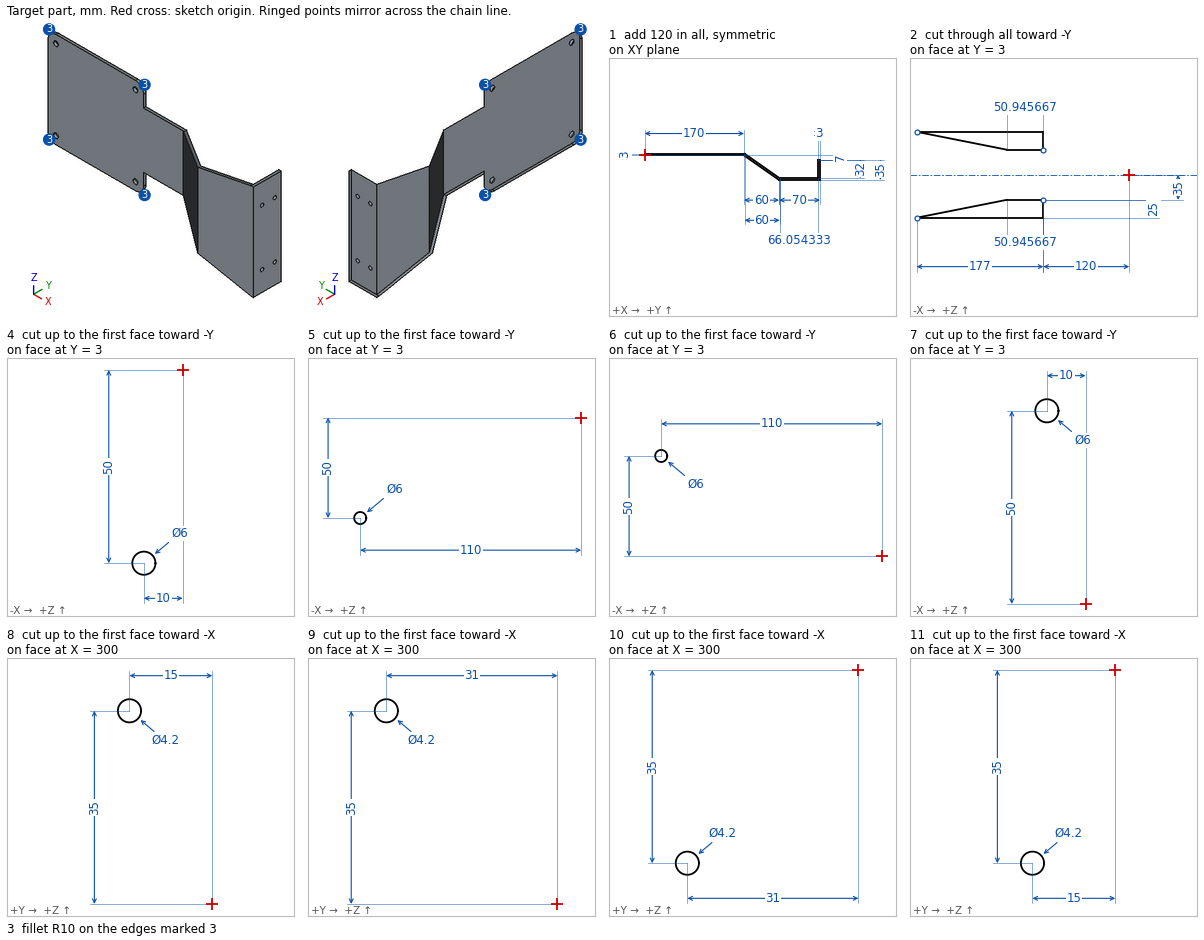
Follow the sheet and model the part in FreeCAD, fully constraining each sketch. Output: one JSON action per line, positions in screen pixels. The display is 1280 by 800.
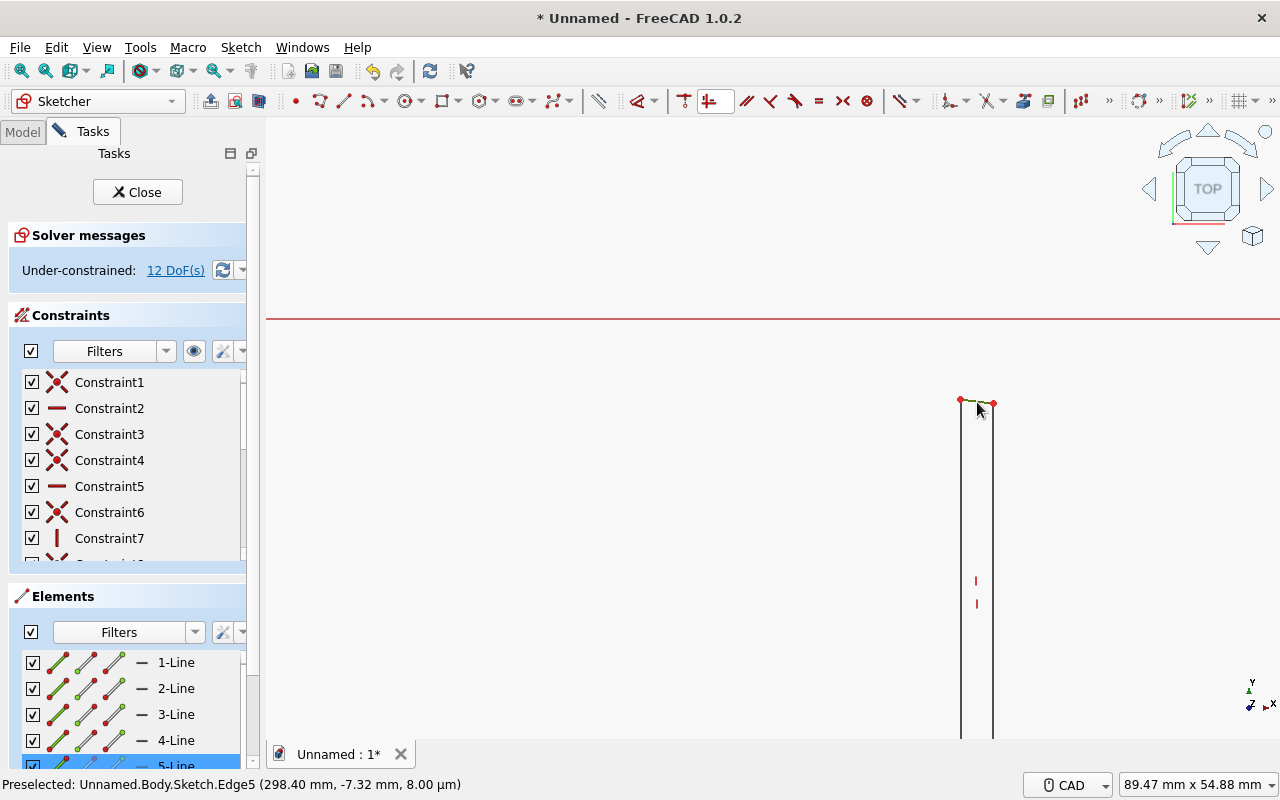
{"action": "left_click", "coordinate": [728, 102]}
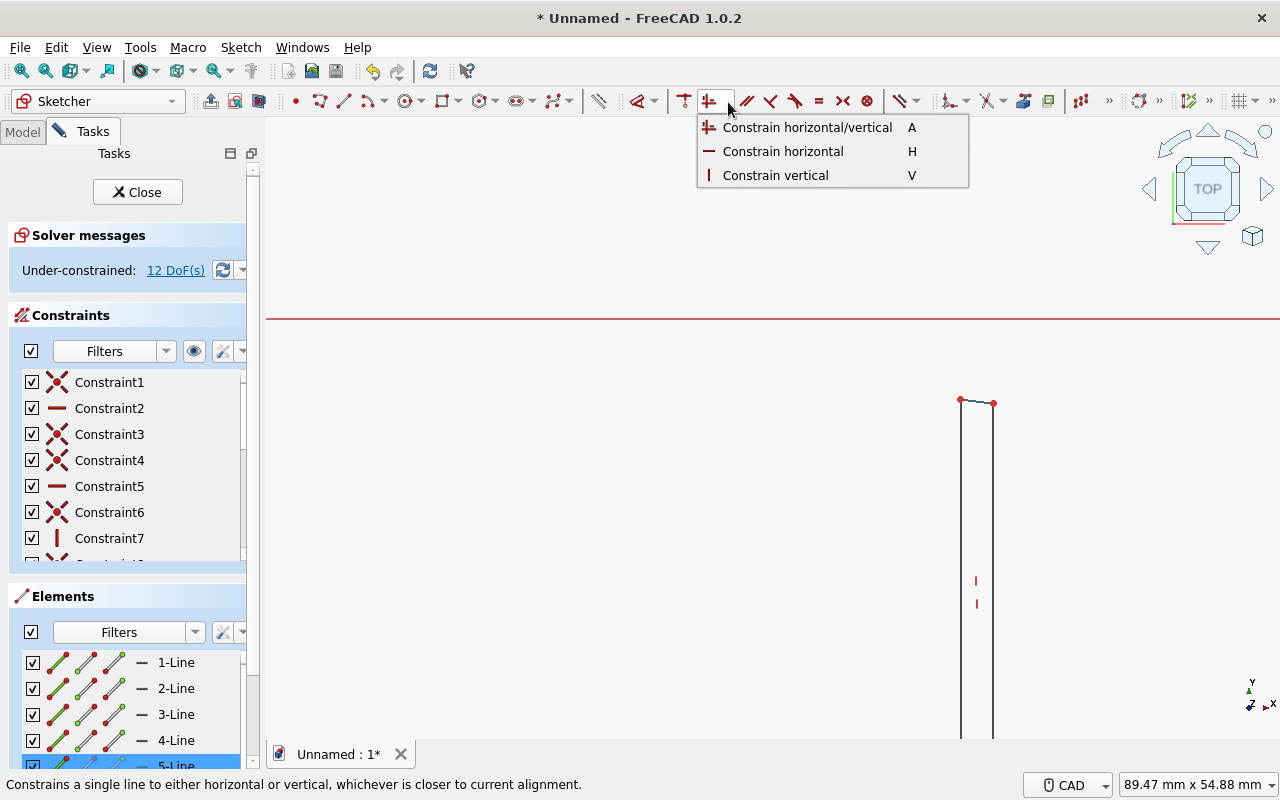
{"action": "left_click", "coordinate": [833, 151]}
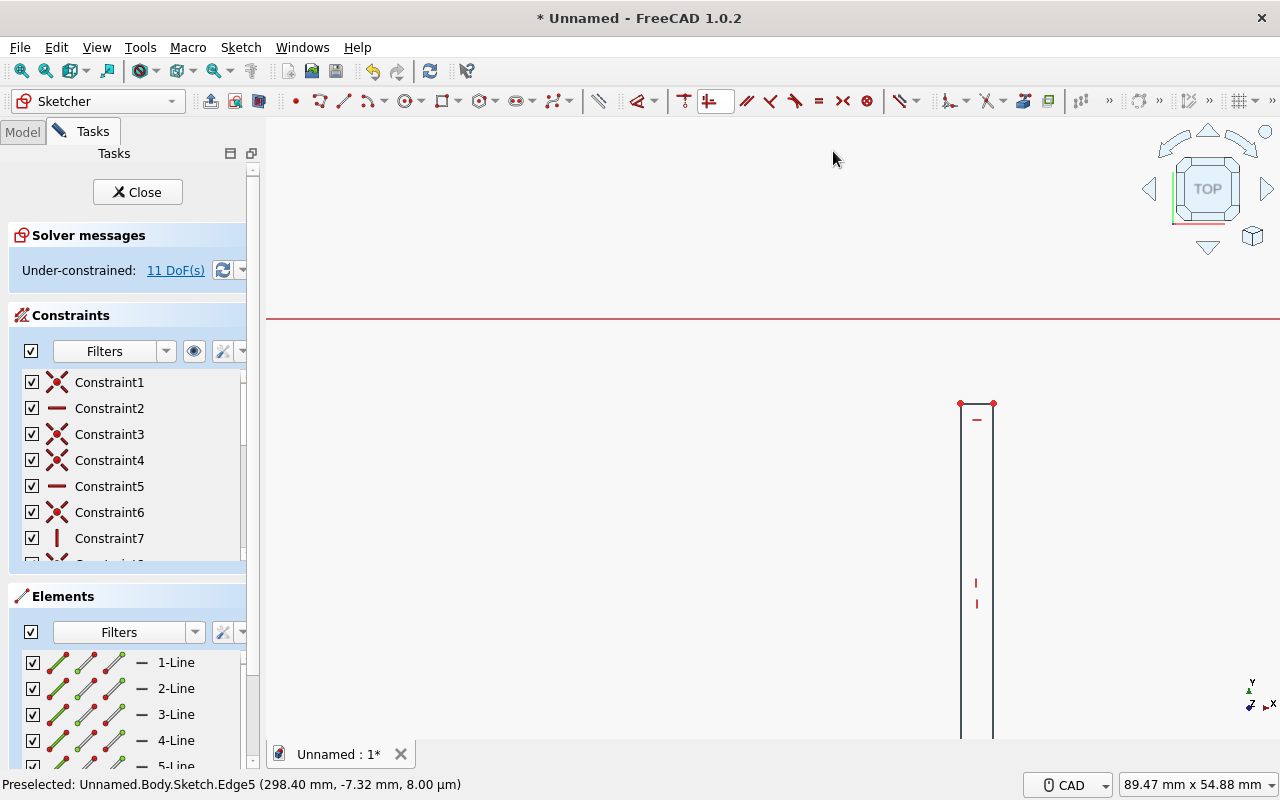
{"action": "scroll", "coordinate": [984, 406], "scroll_direction": "down", "scroll_amount": 9}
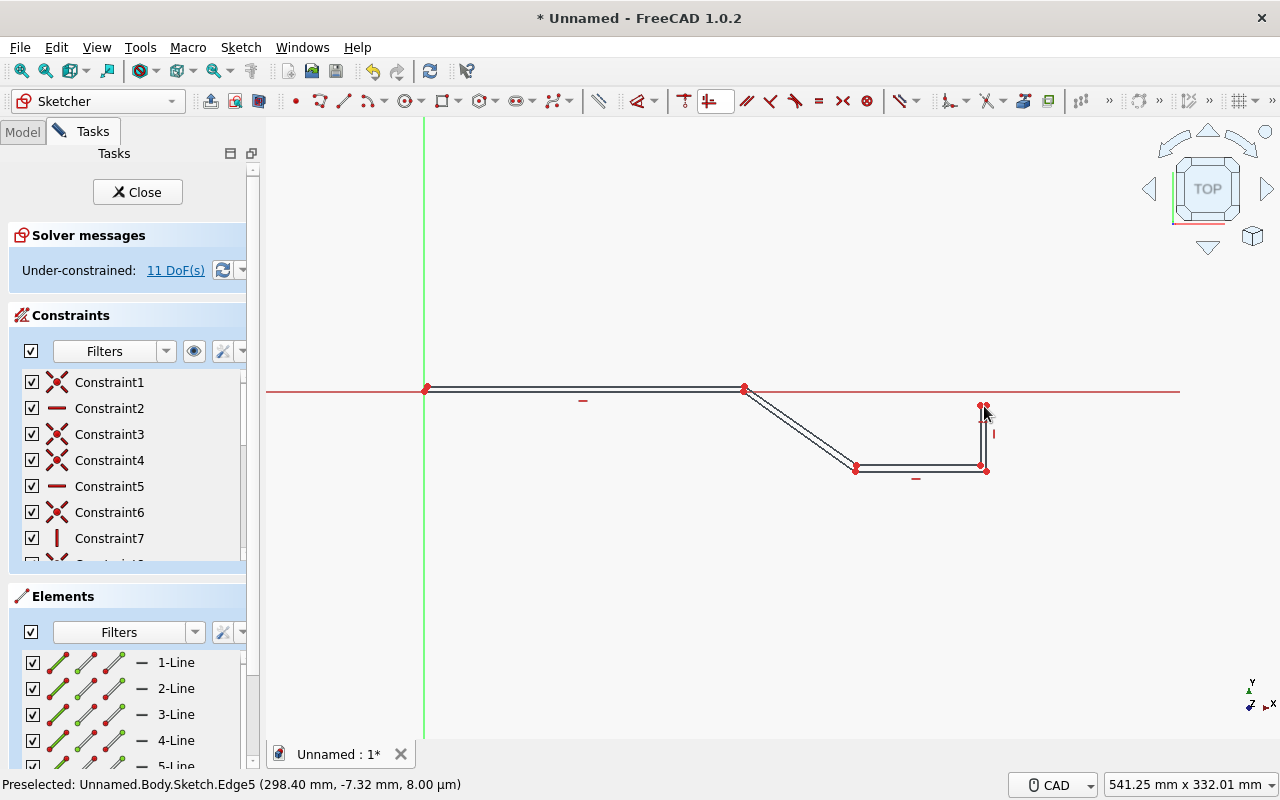
{"action": "scroll", "coordinate": [426, 388], "scroll_direction": "up", "scroll_amount": 11}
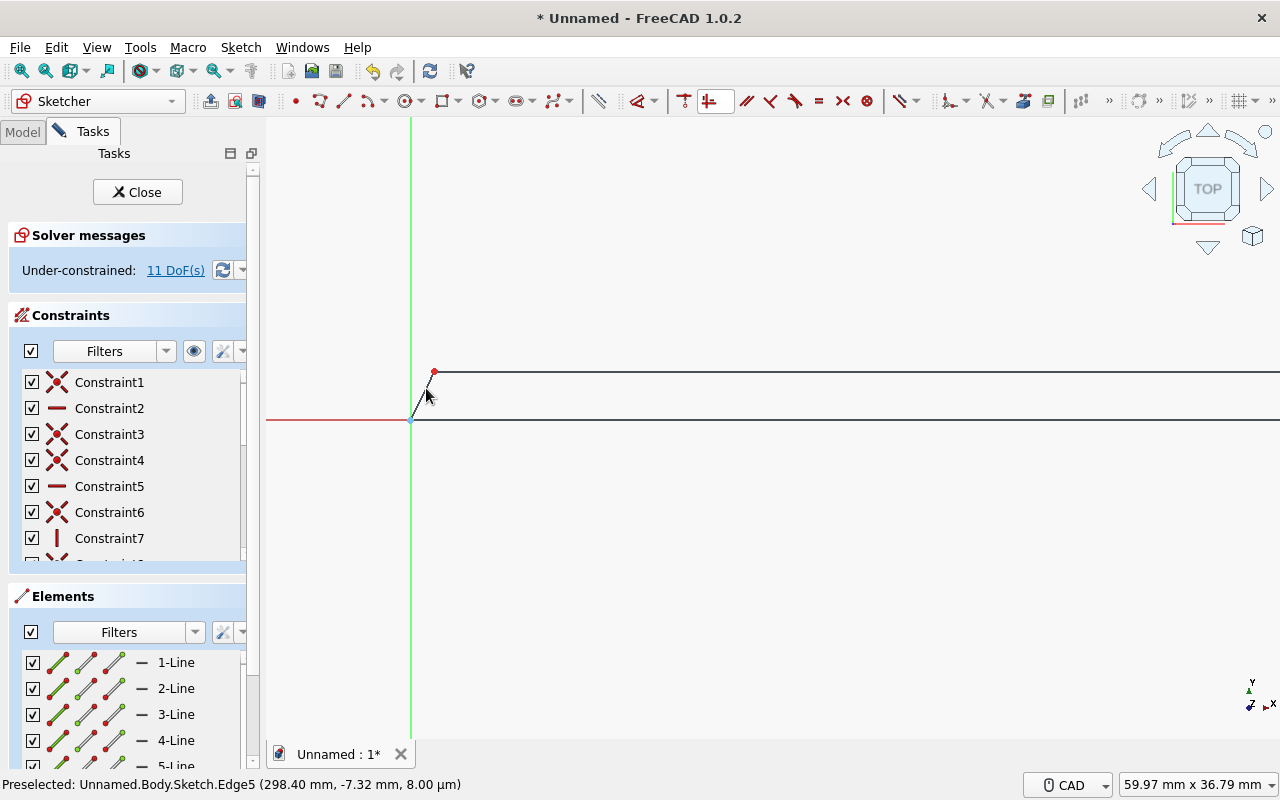
{"action": "left_click", "coordinate": [427, 386]}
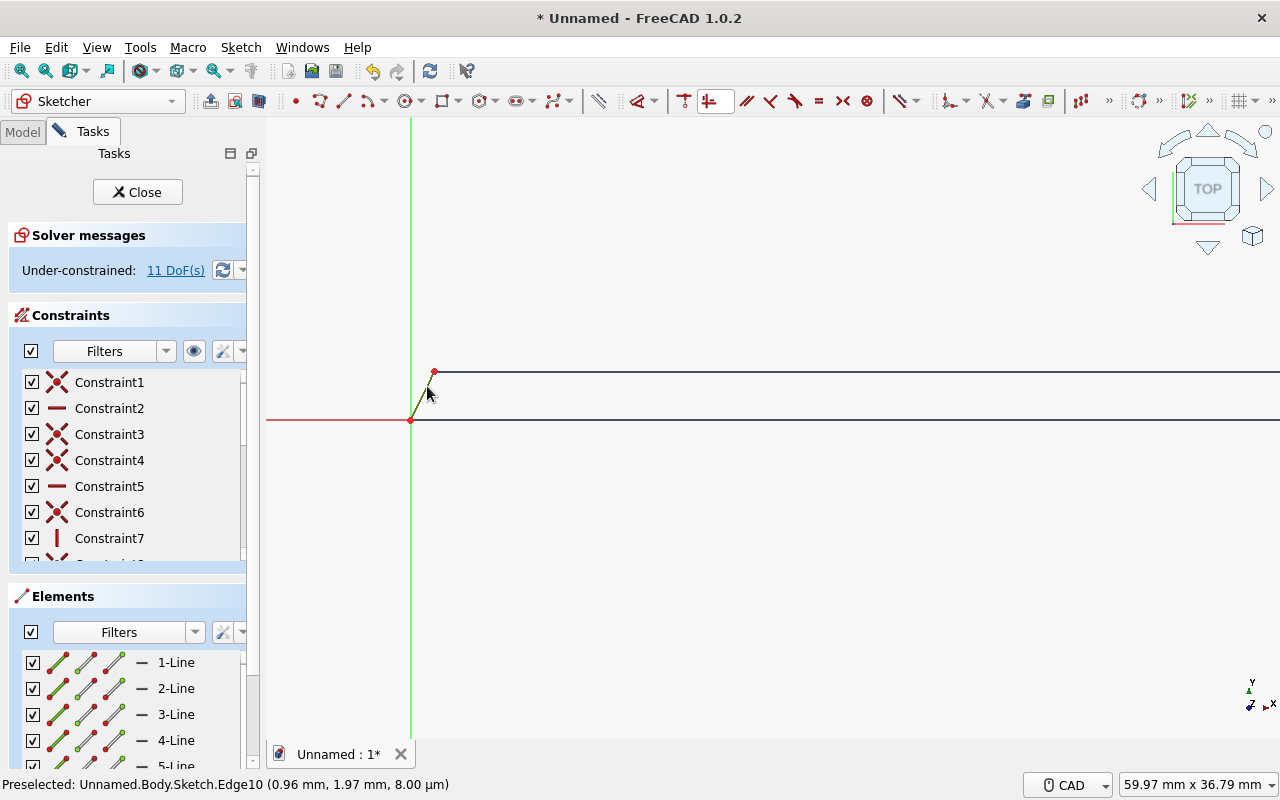
{"action": "left_click", "coordinate": [728, 102]}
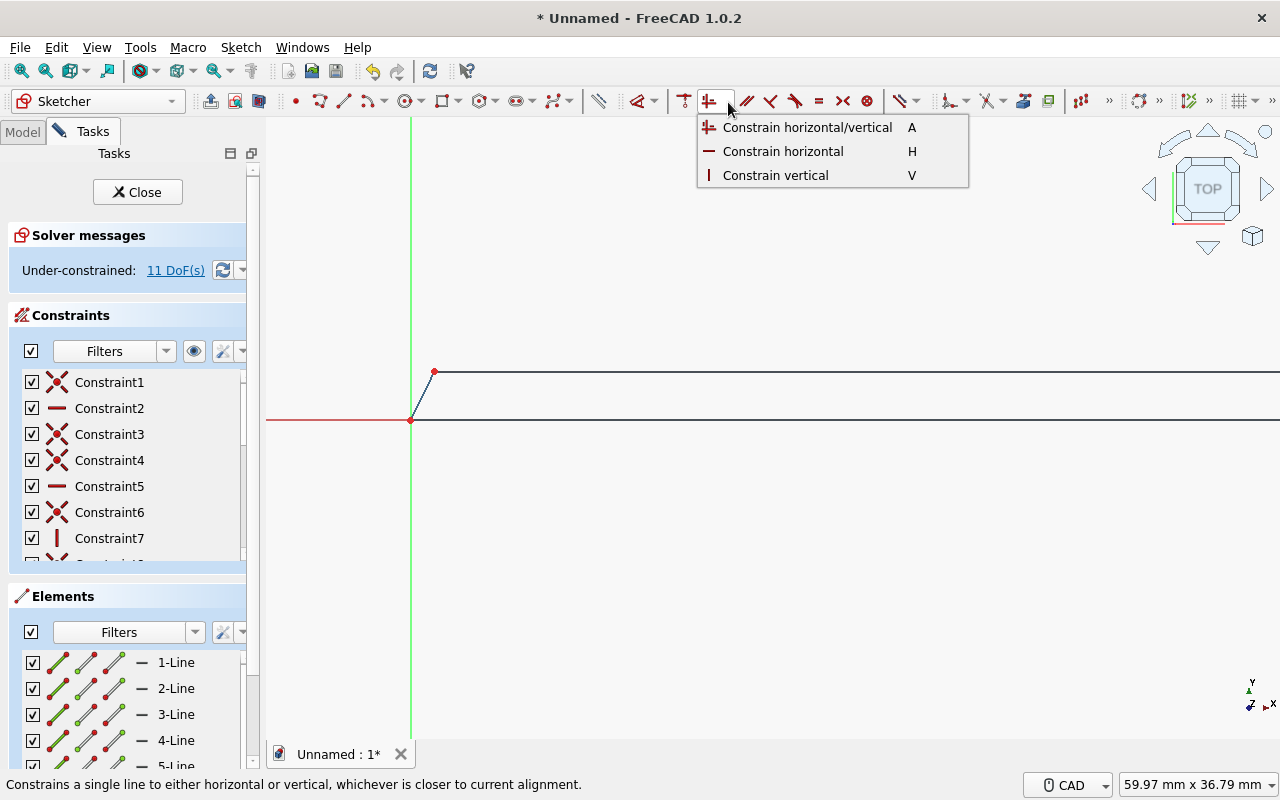
{"action": "left_click", "coordinate": [833, 175]}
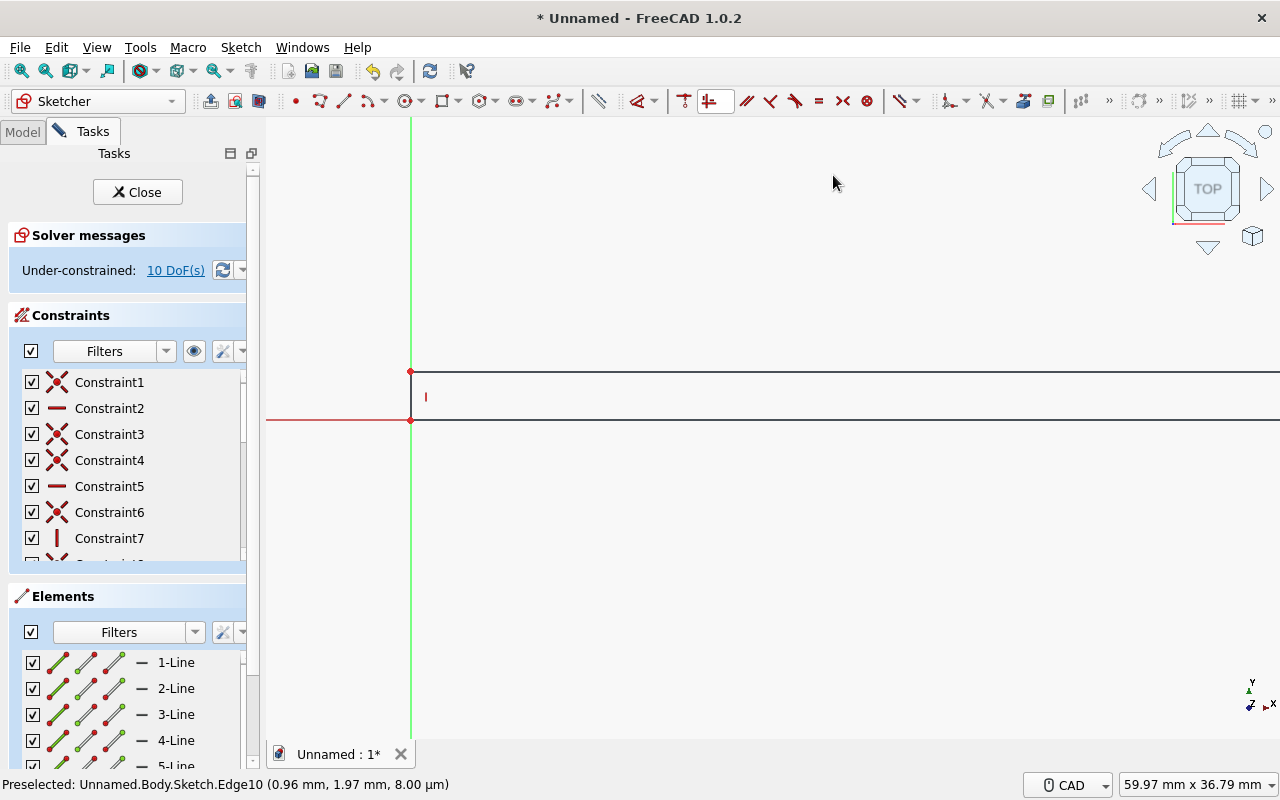
{"action": "left_click", "coordinate": [638, 102]}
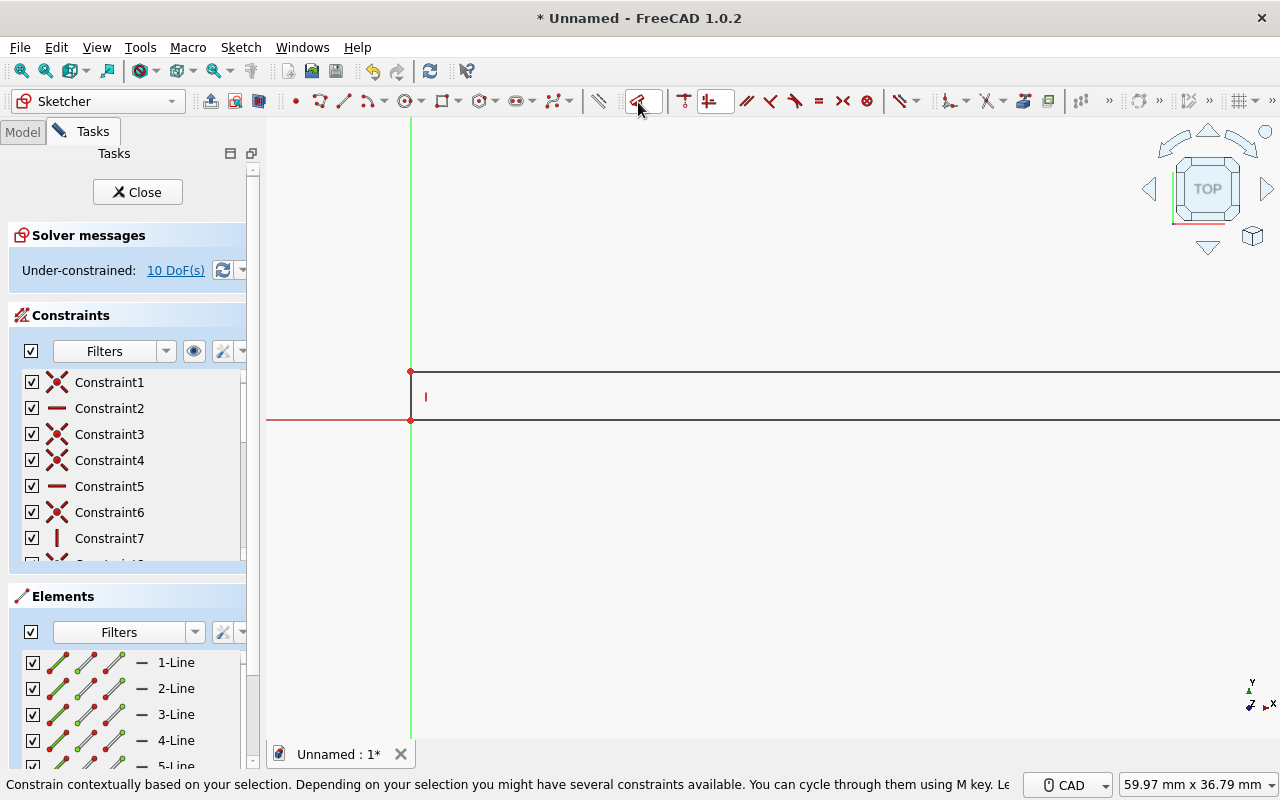
{"action": "scroll", "coordinate": [425, 388], "scroll_direction": "down", "scroll_amount": 11}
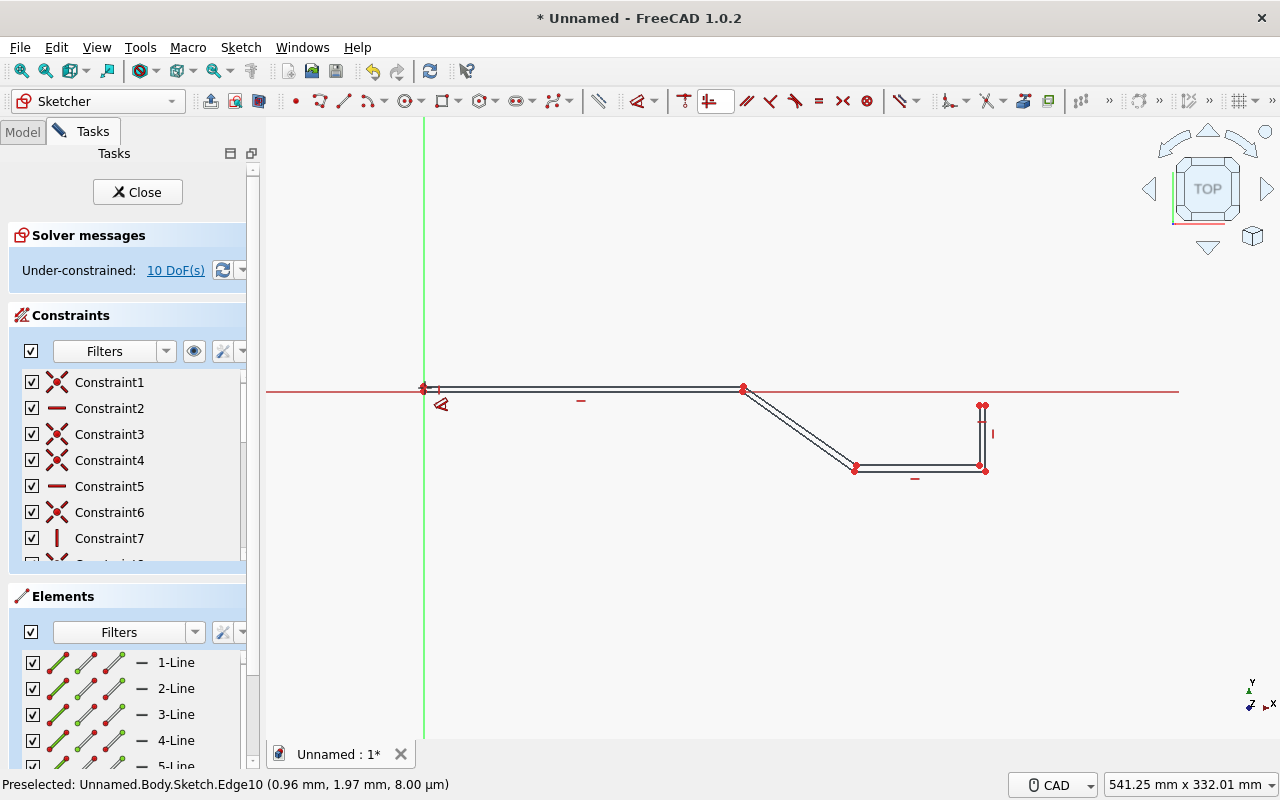
{"action": "scroll", "coordinate": [984, 406], "scroll_direction": "up", "scroll_amount": 11}